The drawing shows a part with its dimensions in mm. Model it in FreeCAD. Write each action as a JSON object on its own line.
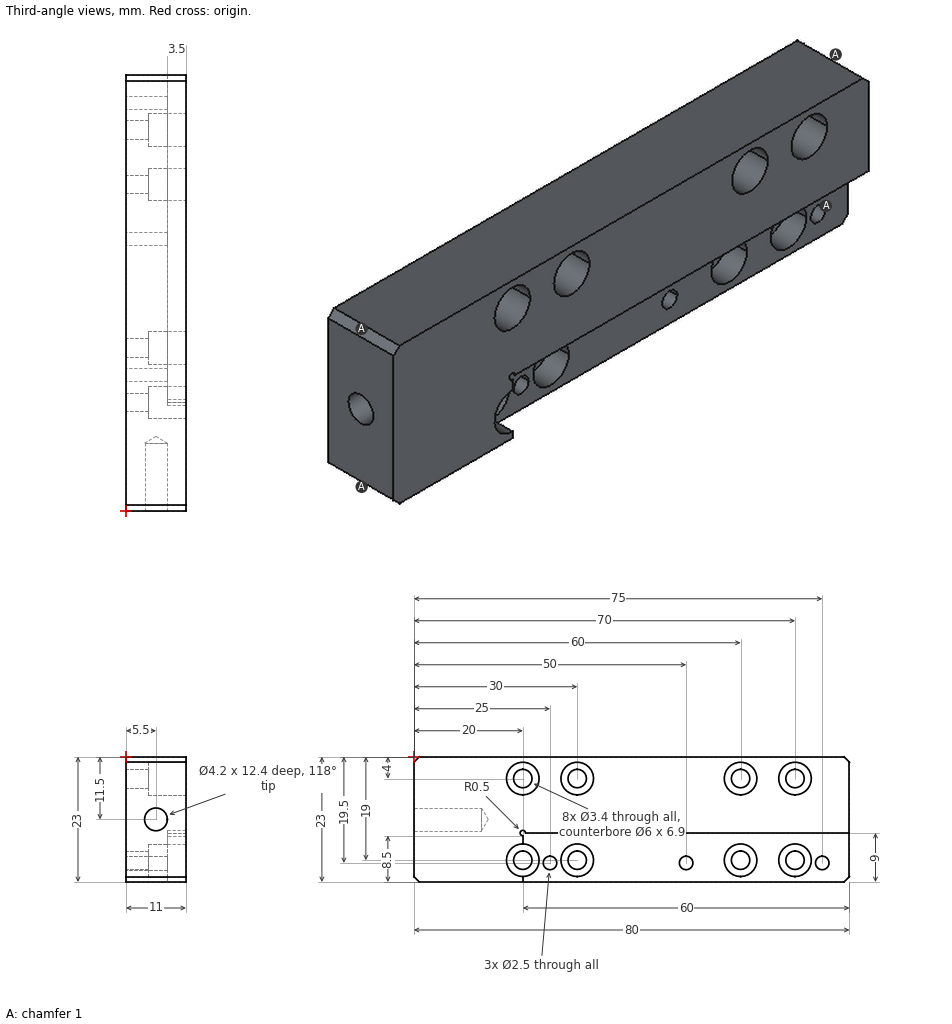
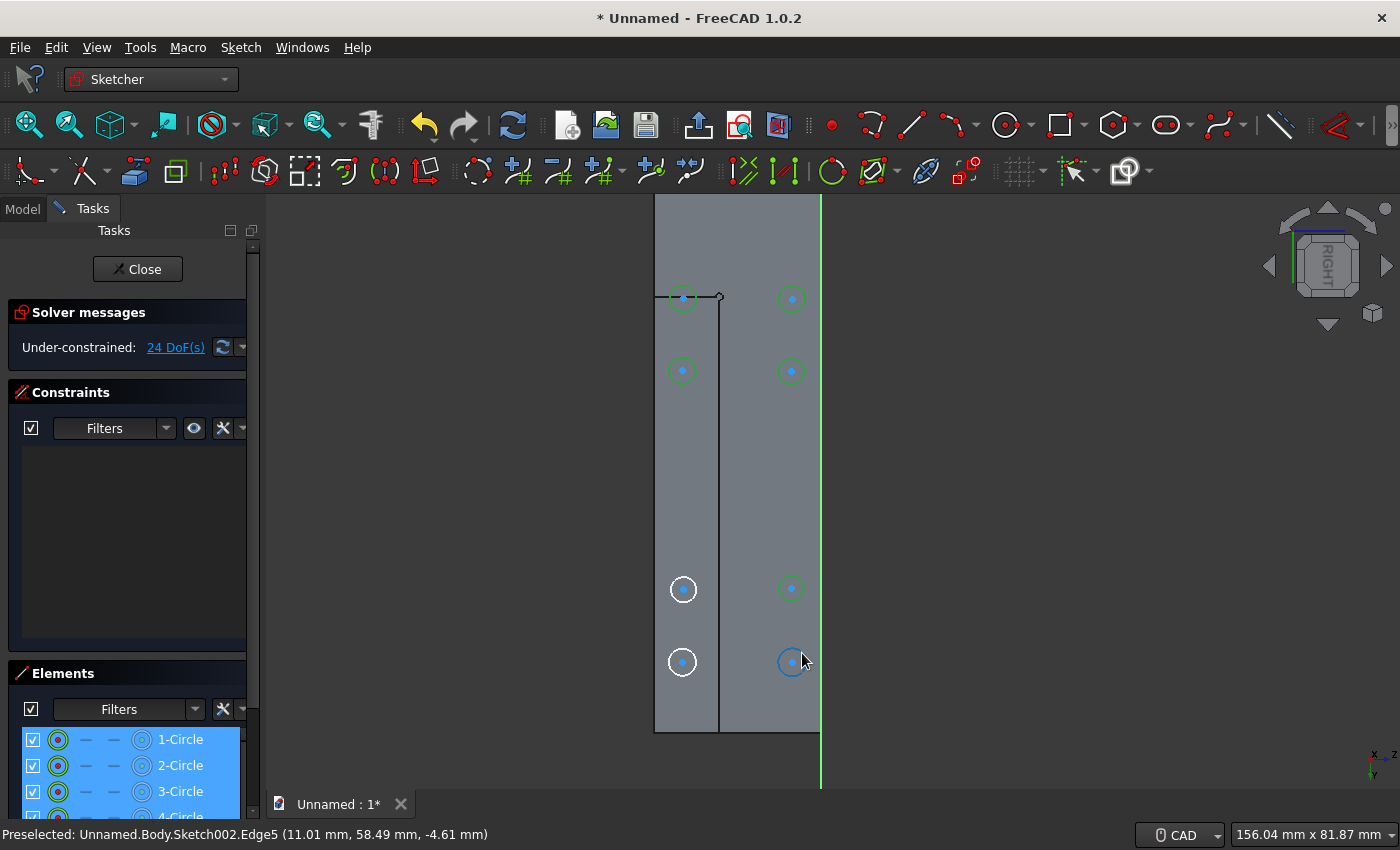
{"action": "left_click", "coordinate": [802, 652]}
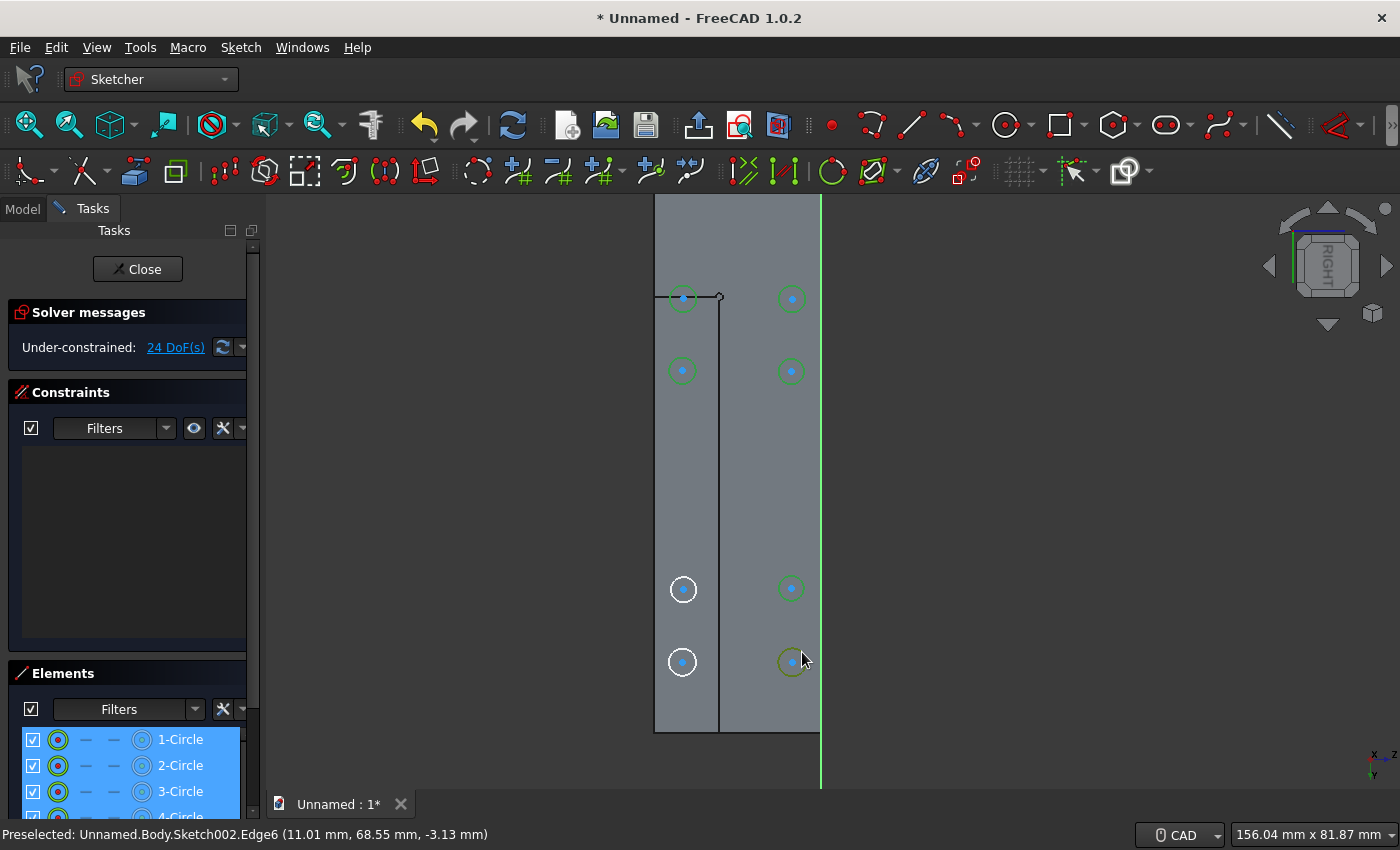
{"action": "left_click", "coordinate": [693, 581]}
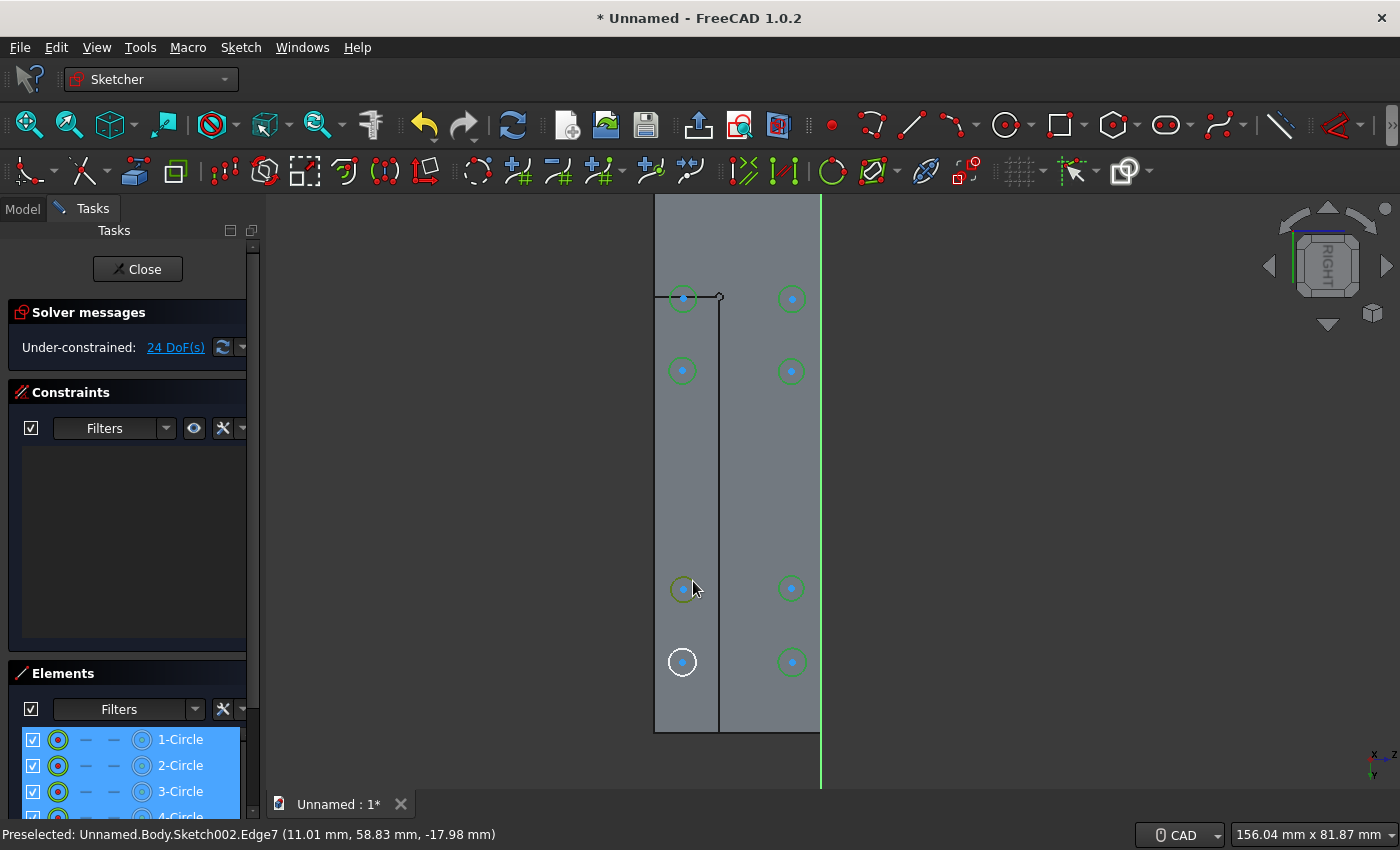
{"action": "left_click", "coordinate": [692, 653]}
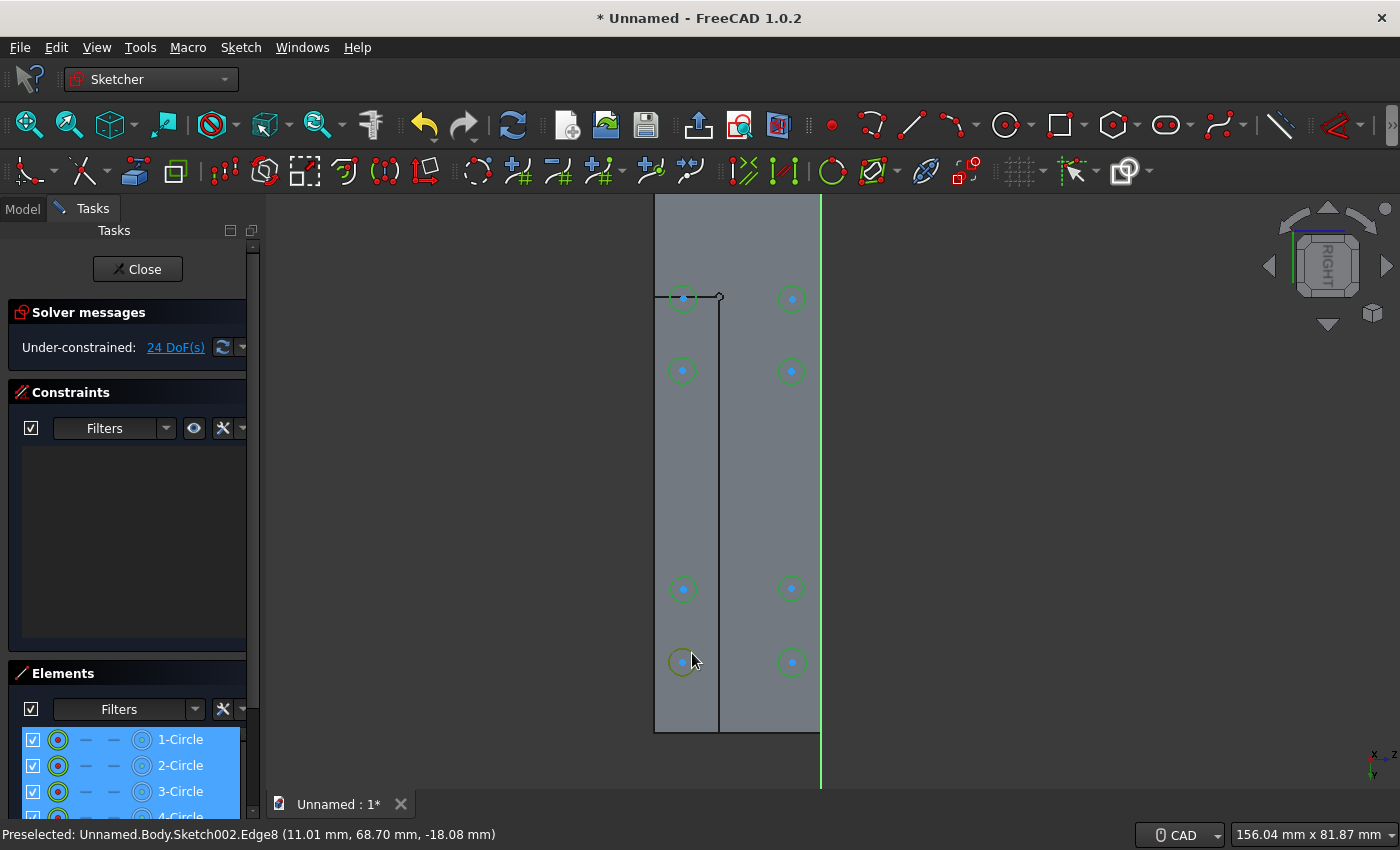
{"action": "key", "text": "e"}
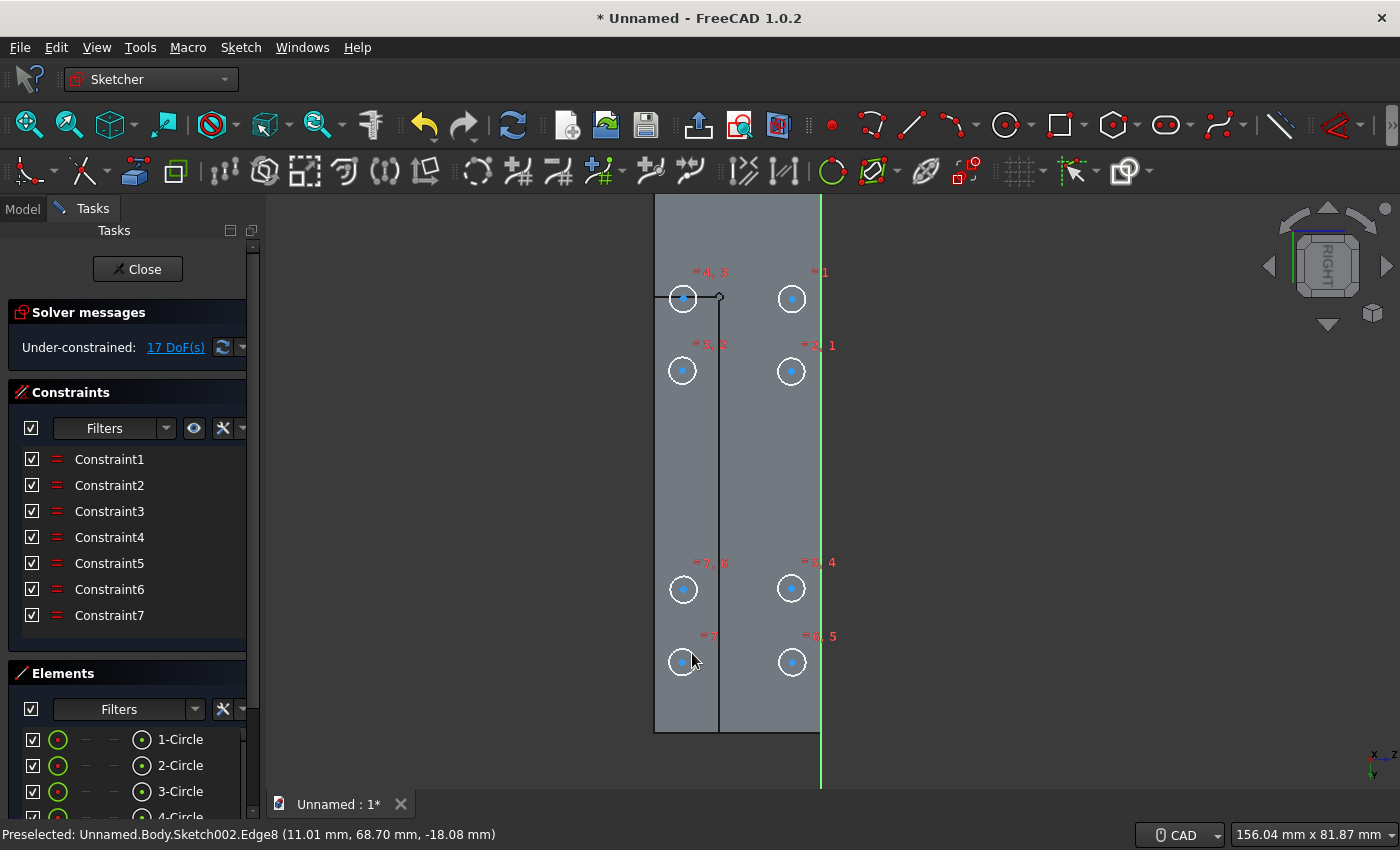
{"action": "left_click", "coordinate": [792, 299]}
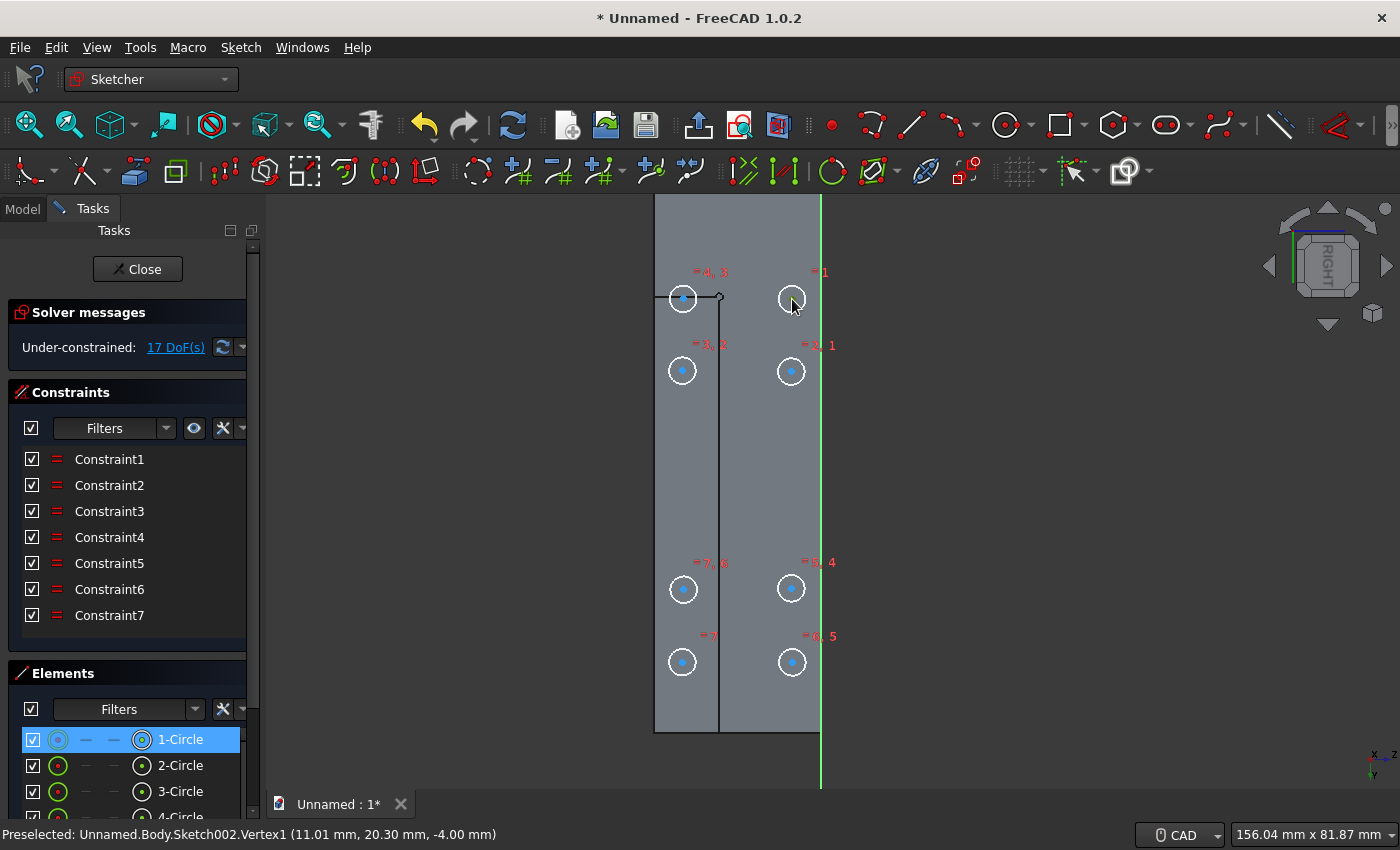
{"action": "left_click", "coordinate": [791, 372]}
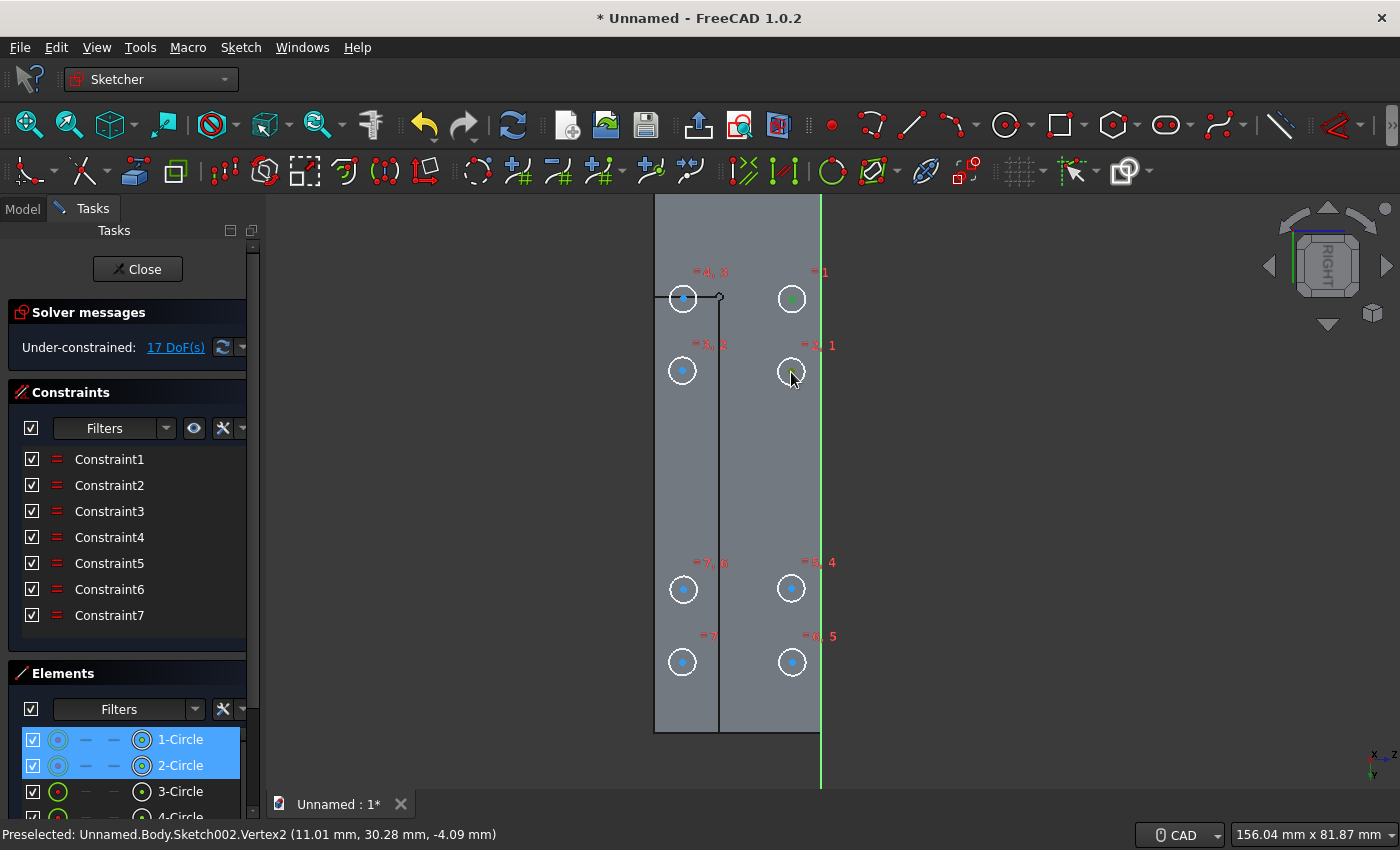
{"action": "key", "text": "v"}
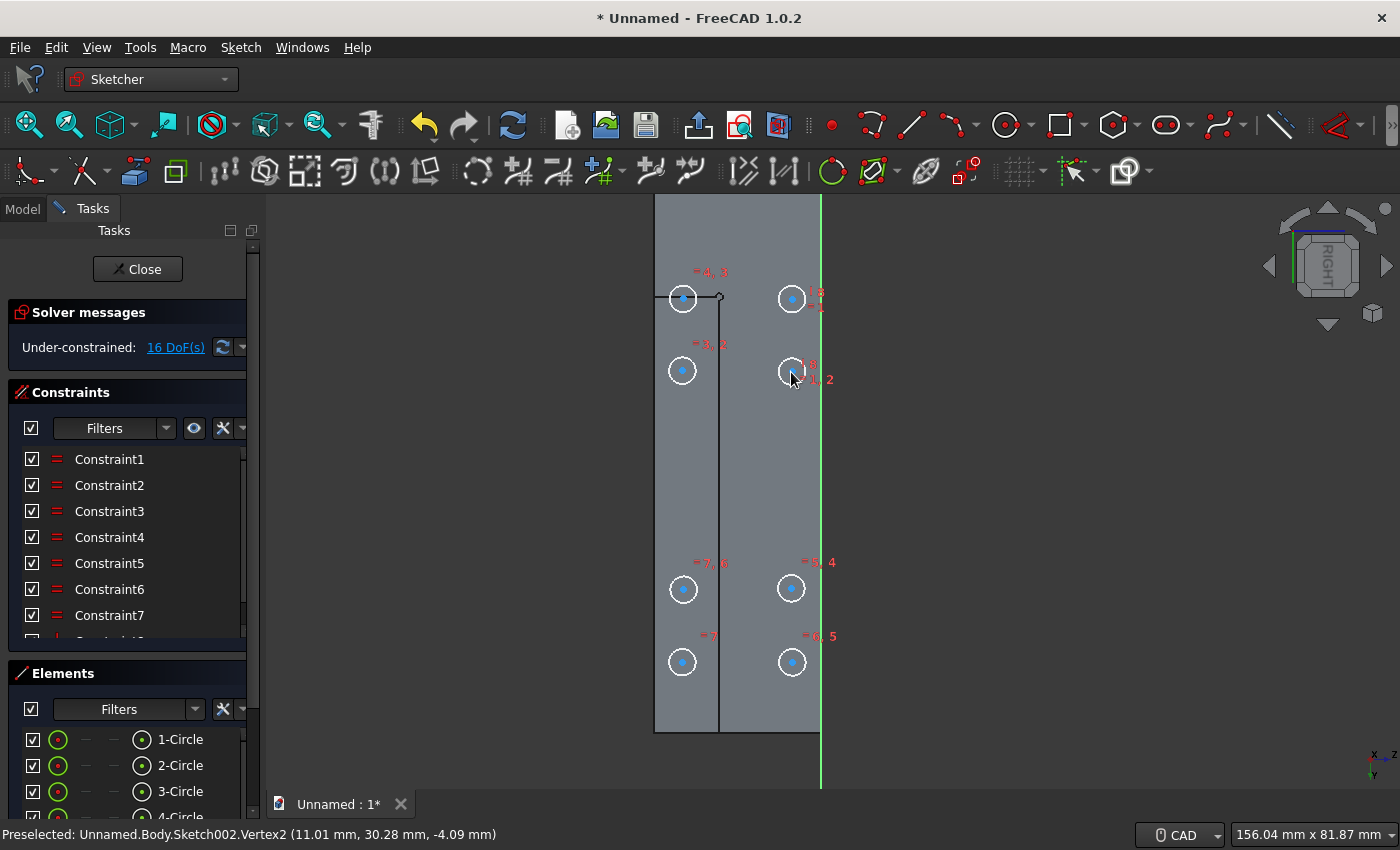
{"action": "left_click", "coordinate": [792, 372]}